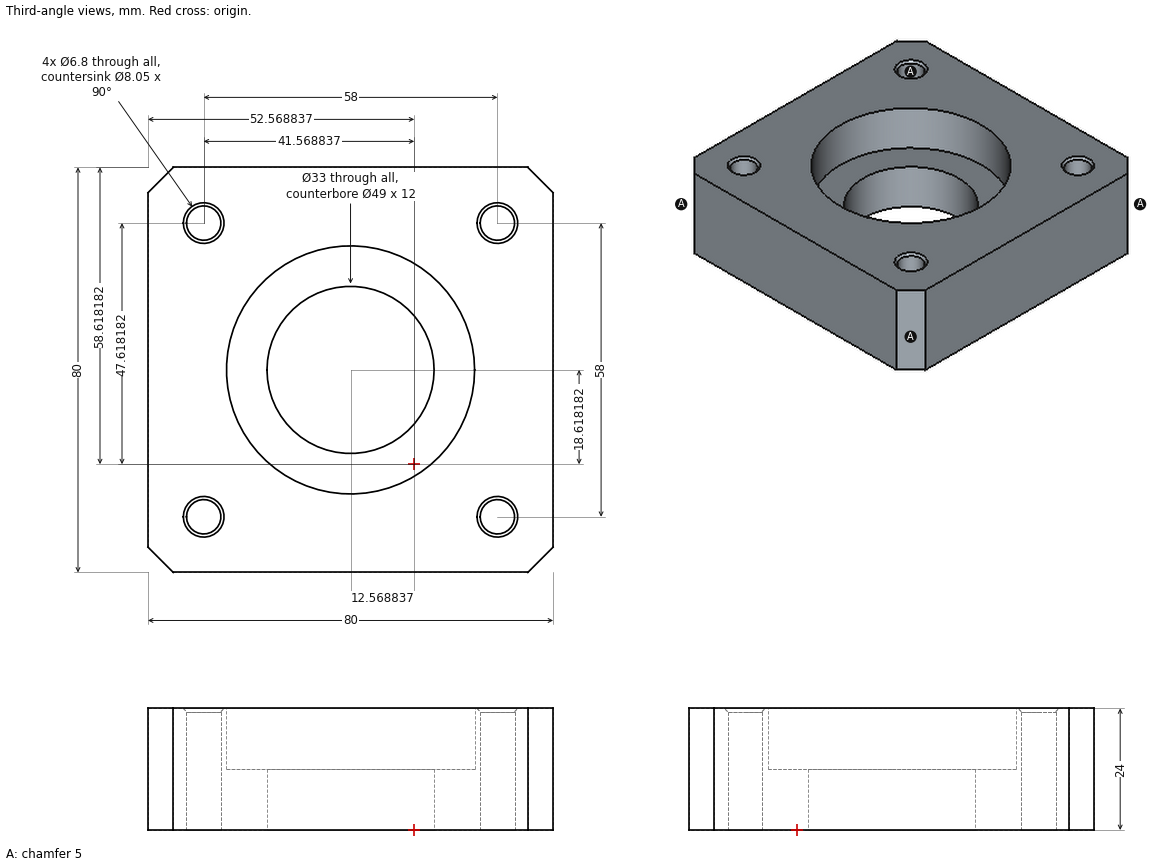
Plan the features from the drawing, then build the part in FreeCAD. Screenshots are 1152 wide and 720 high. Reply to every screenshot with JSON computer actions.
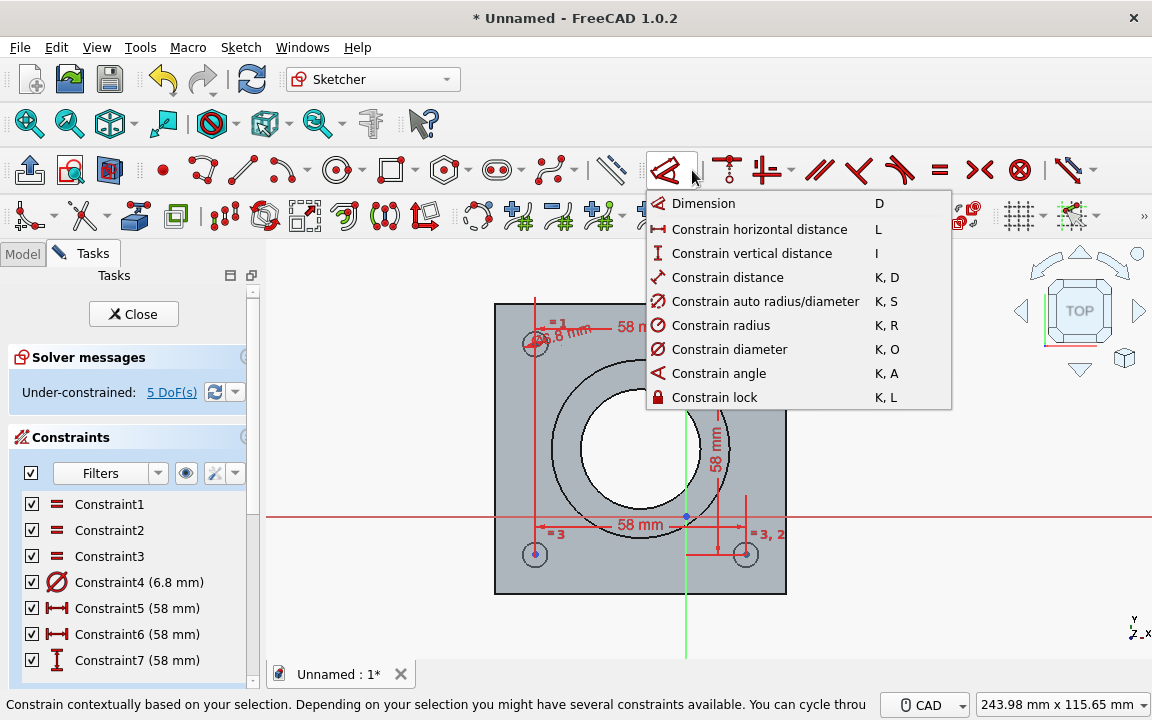
{"action": "left_click", "coordinate": [799, 253]}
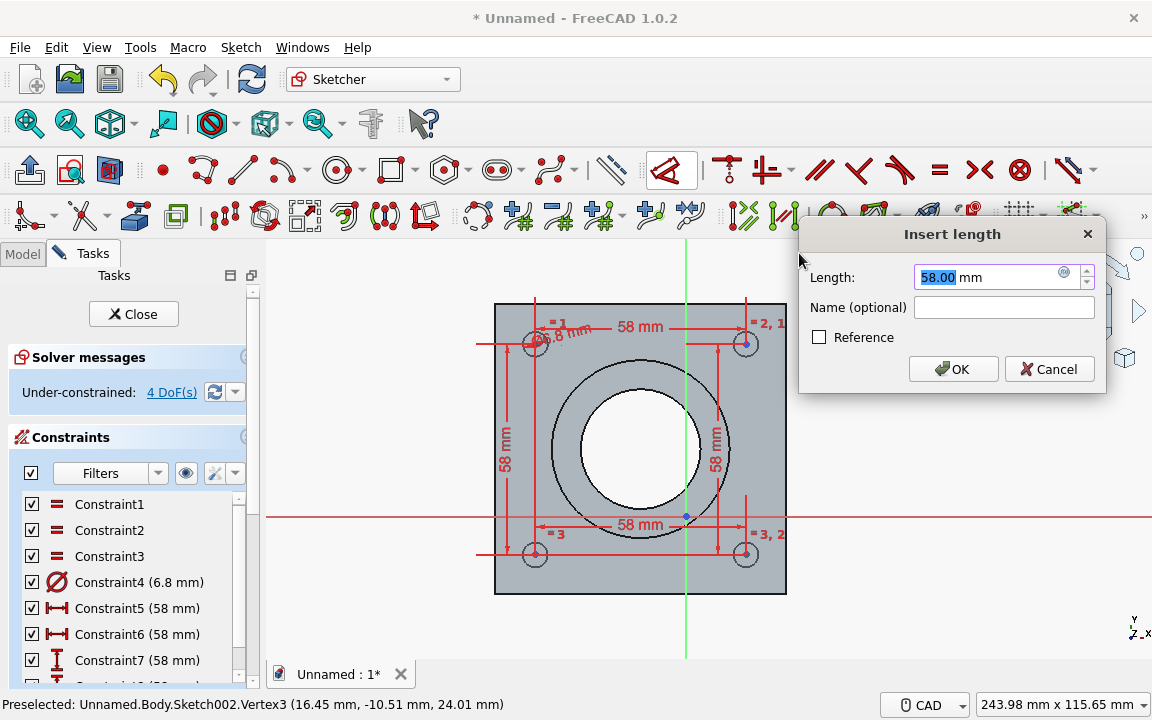
{"action": "type", "text": "58"}
{"action": "key", "text": "Return"}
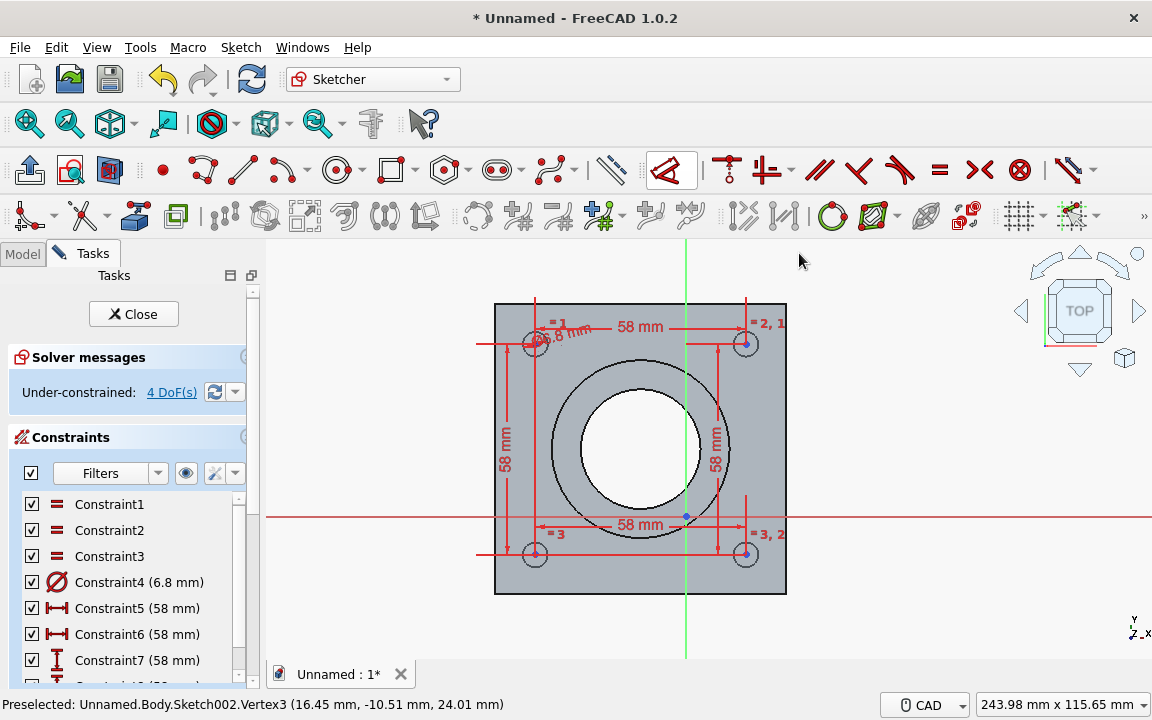
{"action": "left_click", "coordinate": [746, 555]}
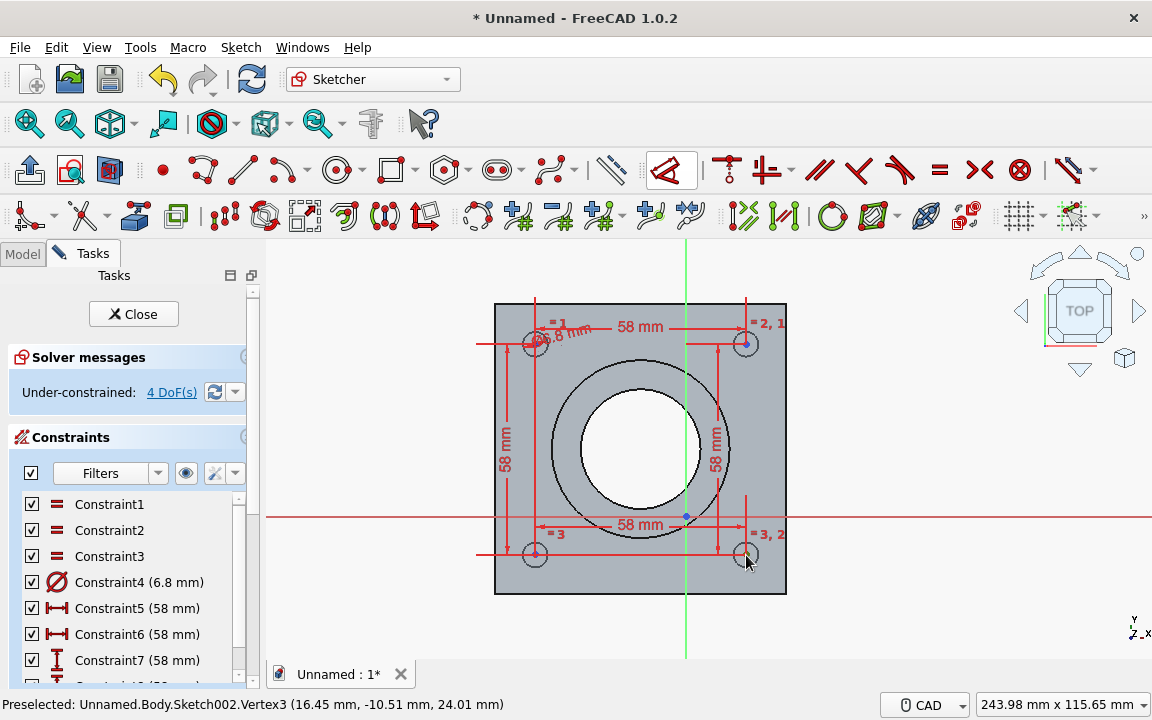
{"action": "left_click", "coordinate": [535, 555]}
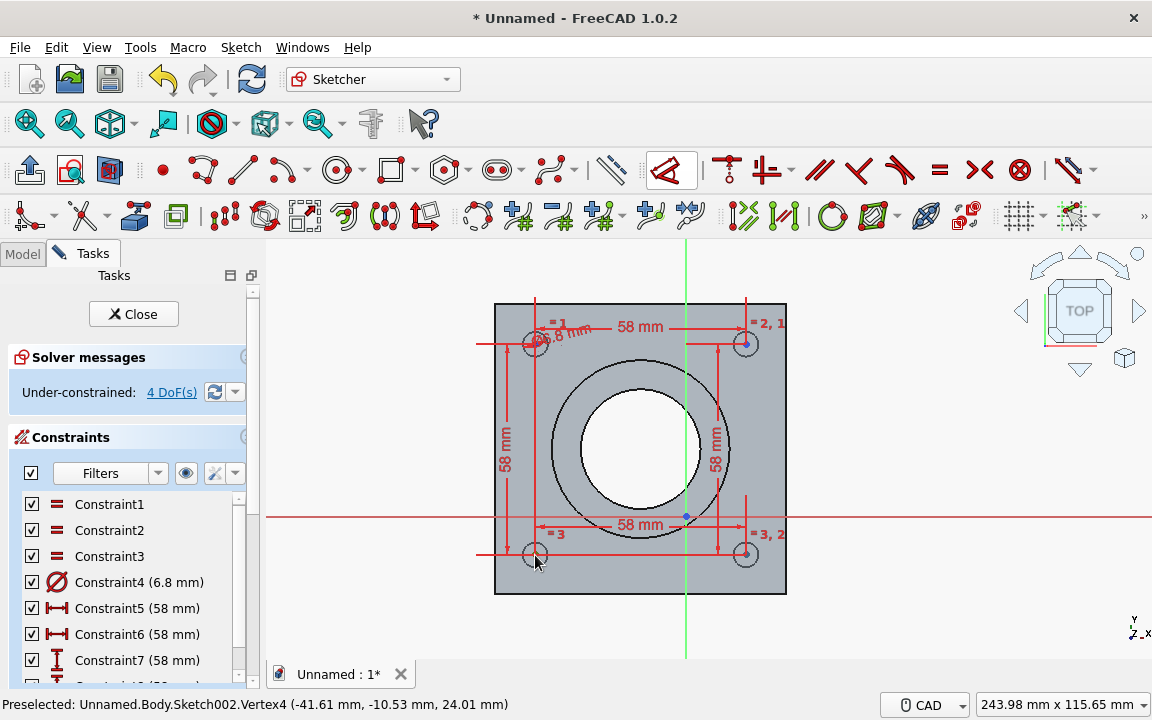
{"action": "key", "text": "l"}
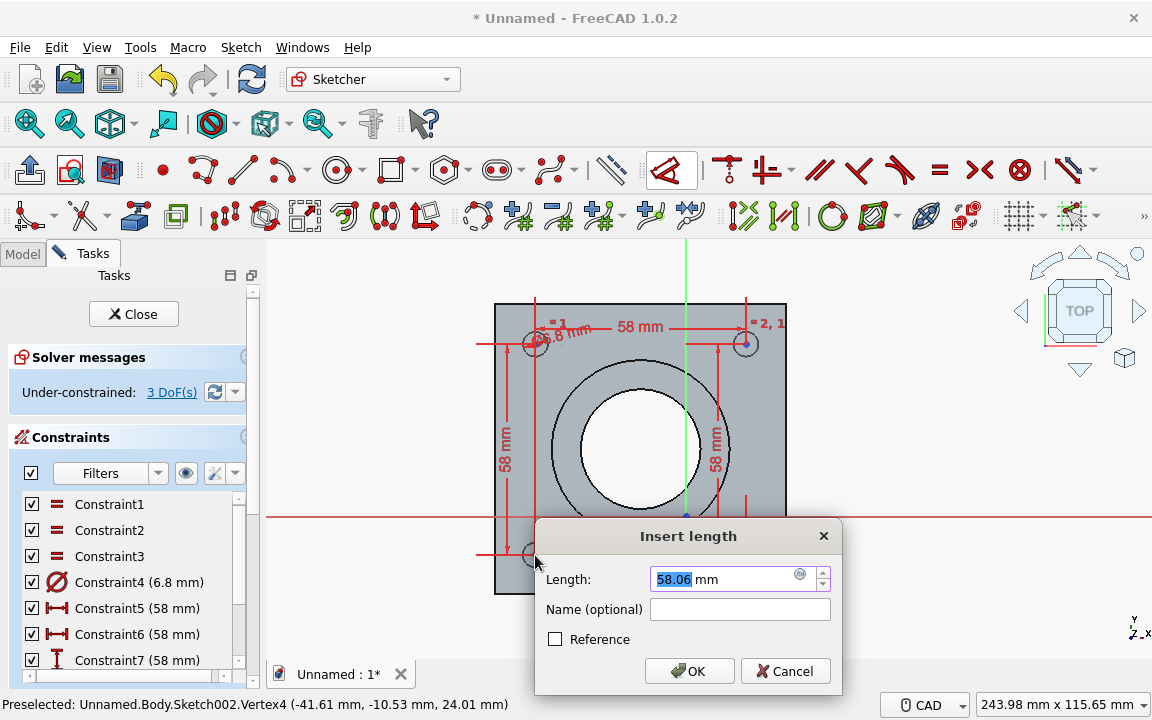
{"action": "type", "text": "58"}
{"action": "key", "text": "Return"}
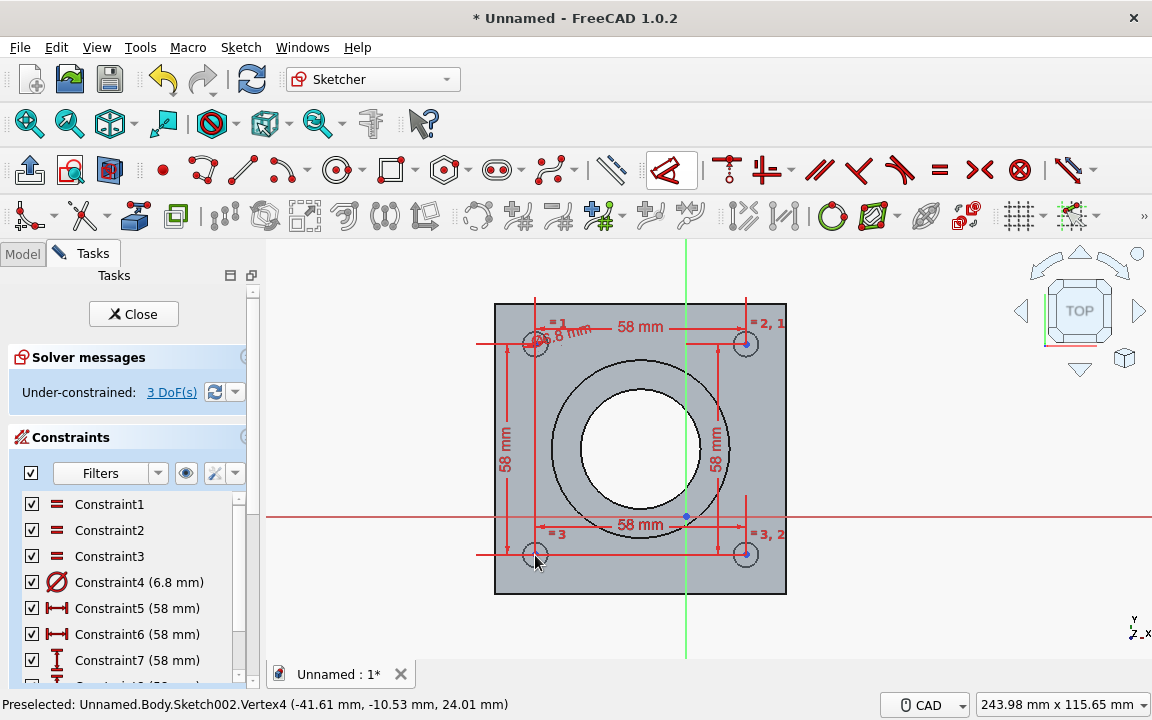
{"action": "left_click", "coordinate": [535, 344]}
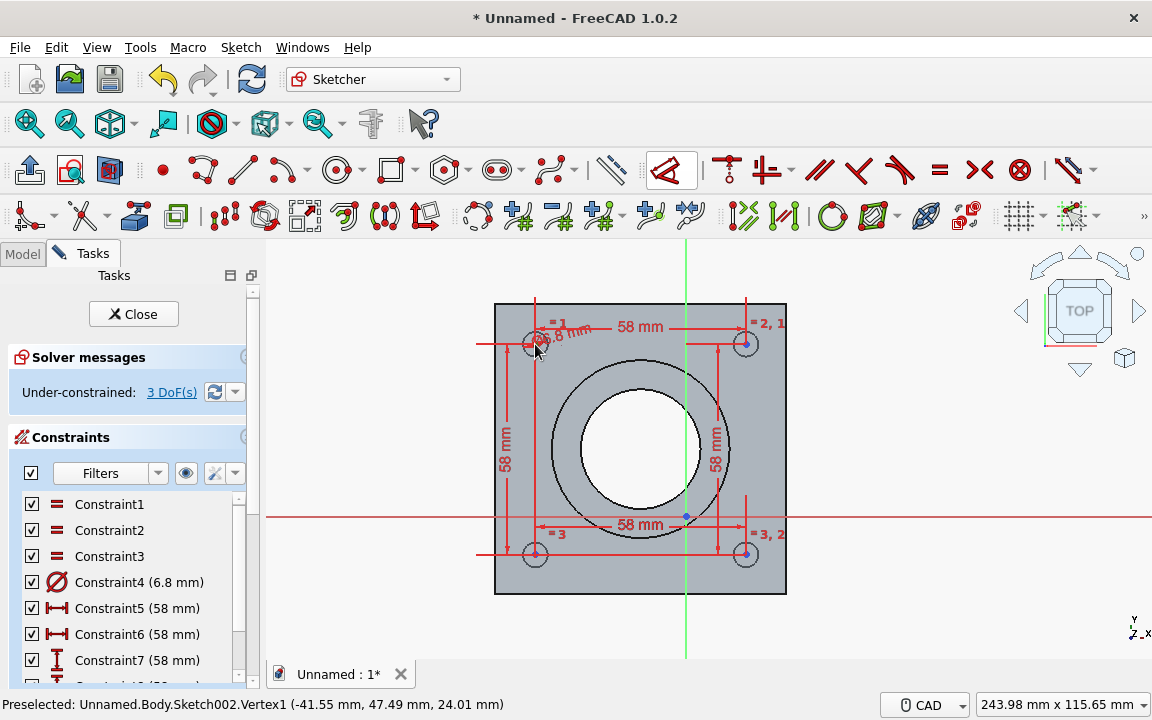
{"action": "left_click", "coordinate": [535, 555]}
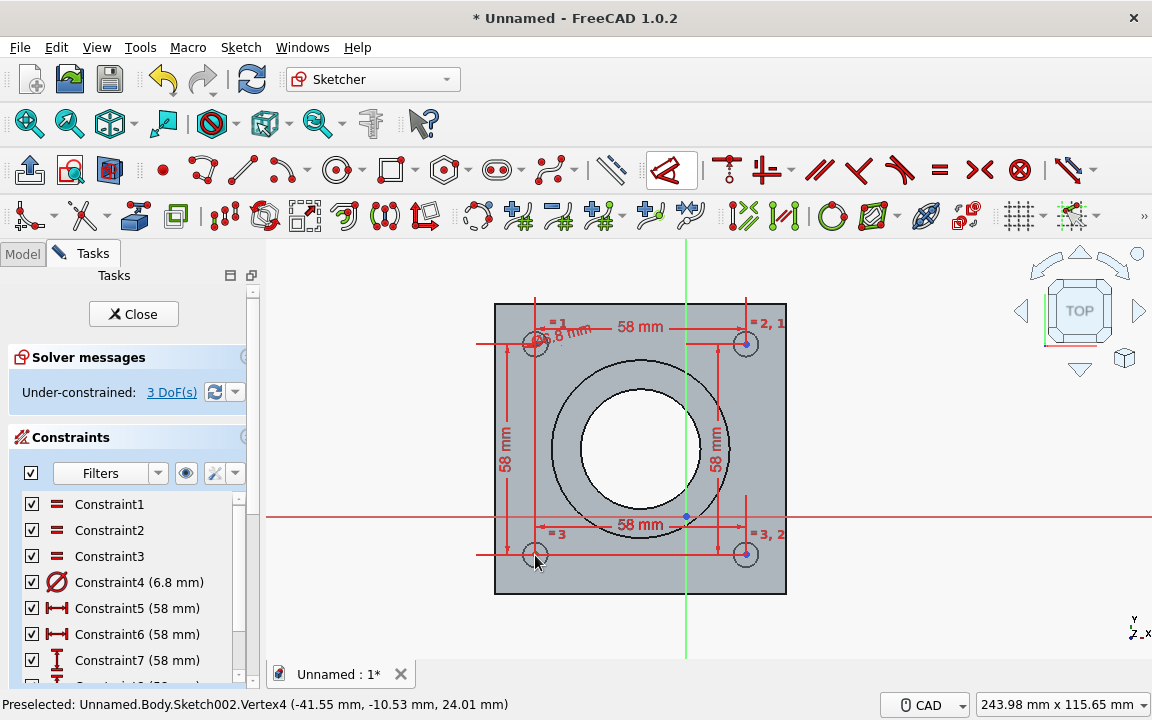
{"action": "left_click", "coordinate": [692, 170]}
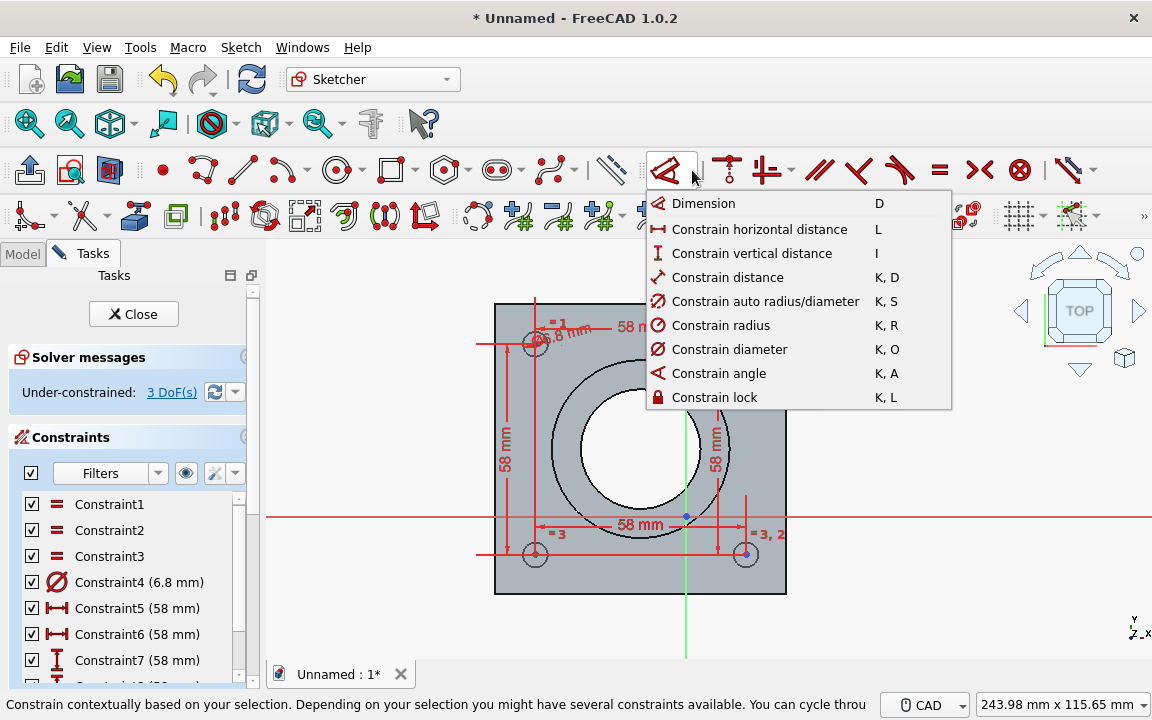
{"action": "left_click", "coordinate": [799, 253]}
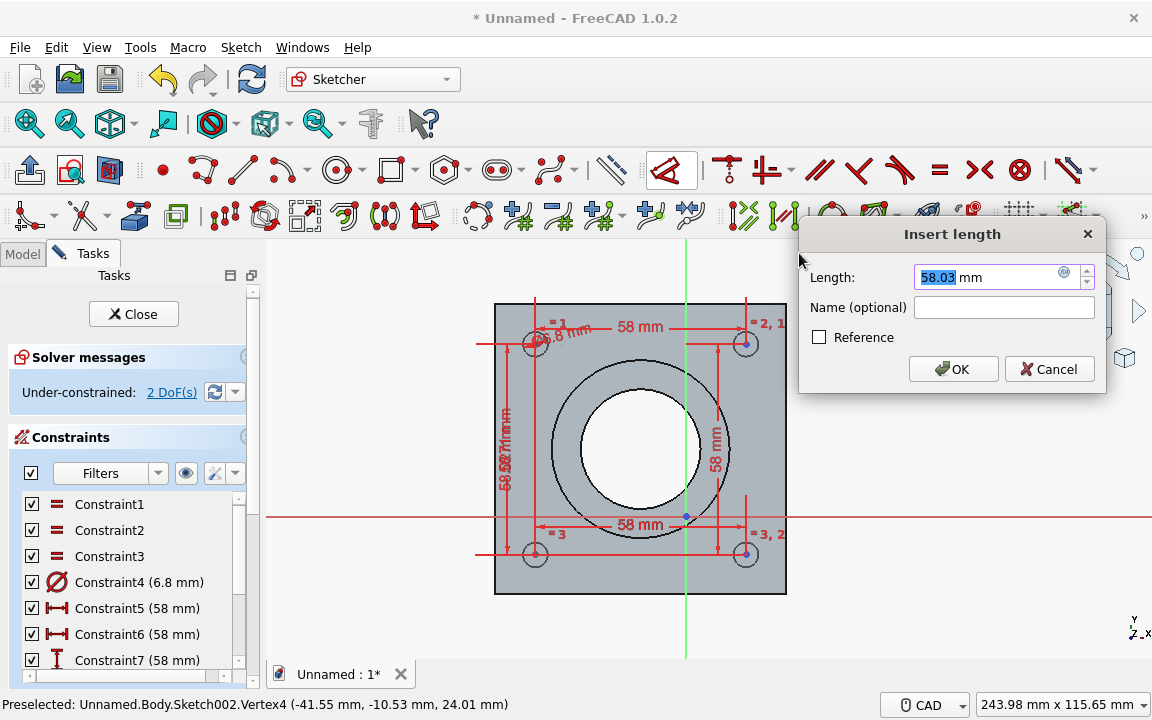
{"action": "type", "text": "58"}
{"action": "key", "text": "Return"}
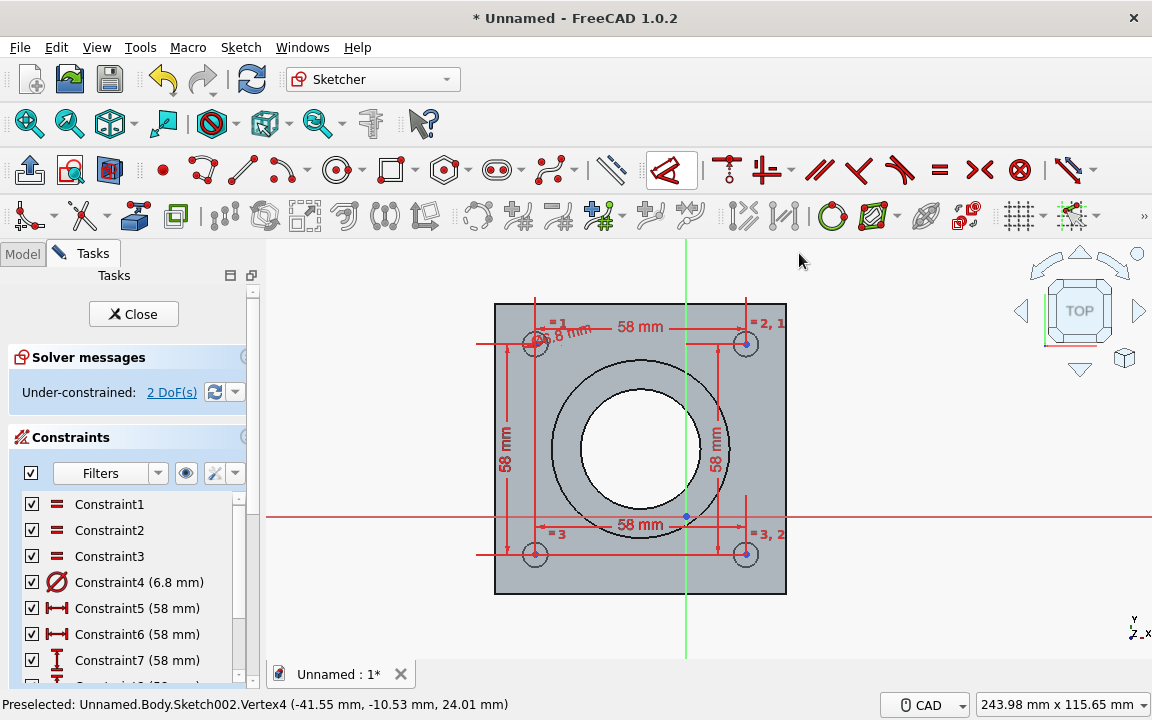
{"action": "left_click", "coordinate": [535, 344]}